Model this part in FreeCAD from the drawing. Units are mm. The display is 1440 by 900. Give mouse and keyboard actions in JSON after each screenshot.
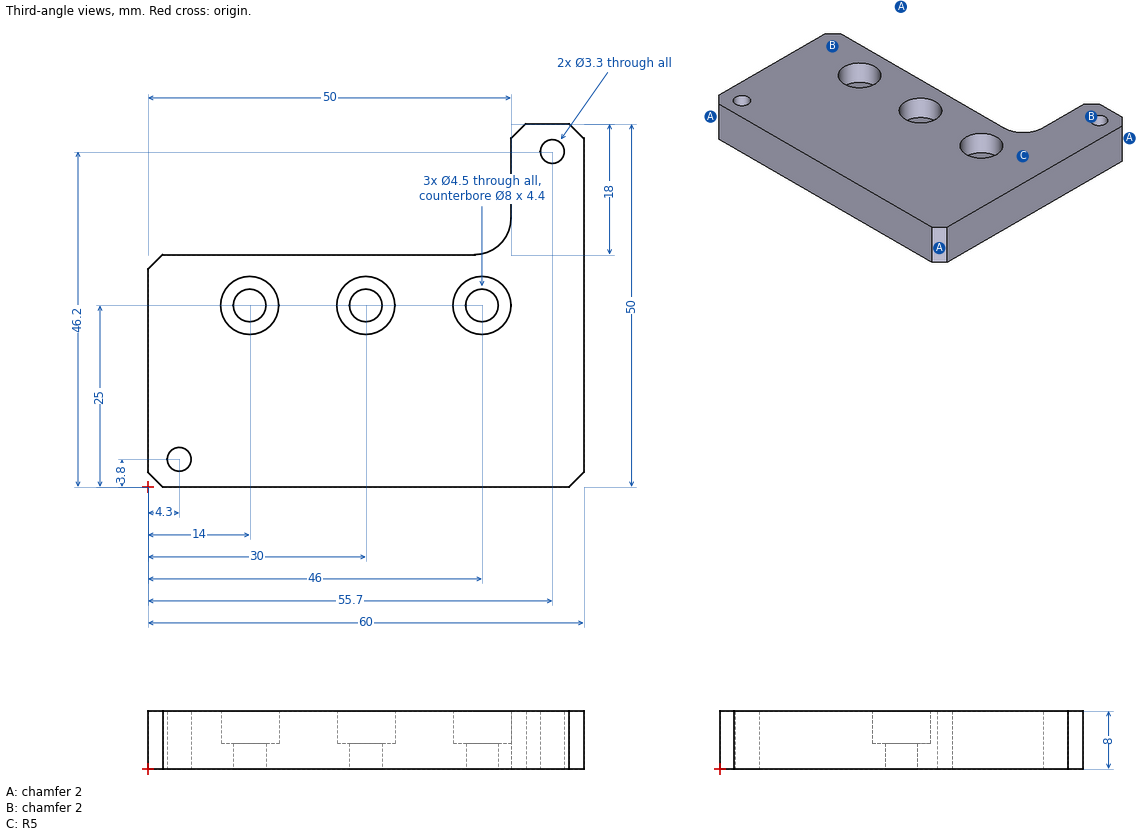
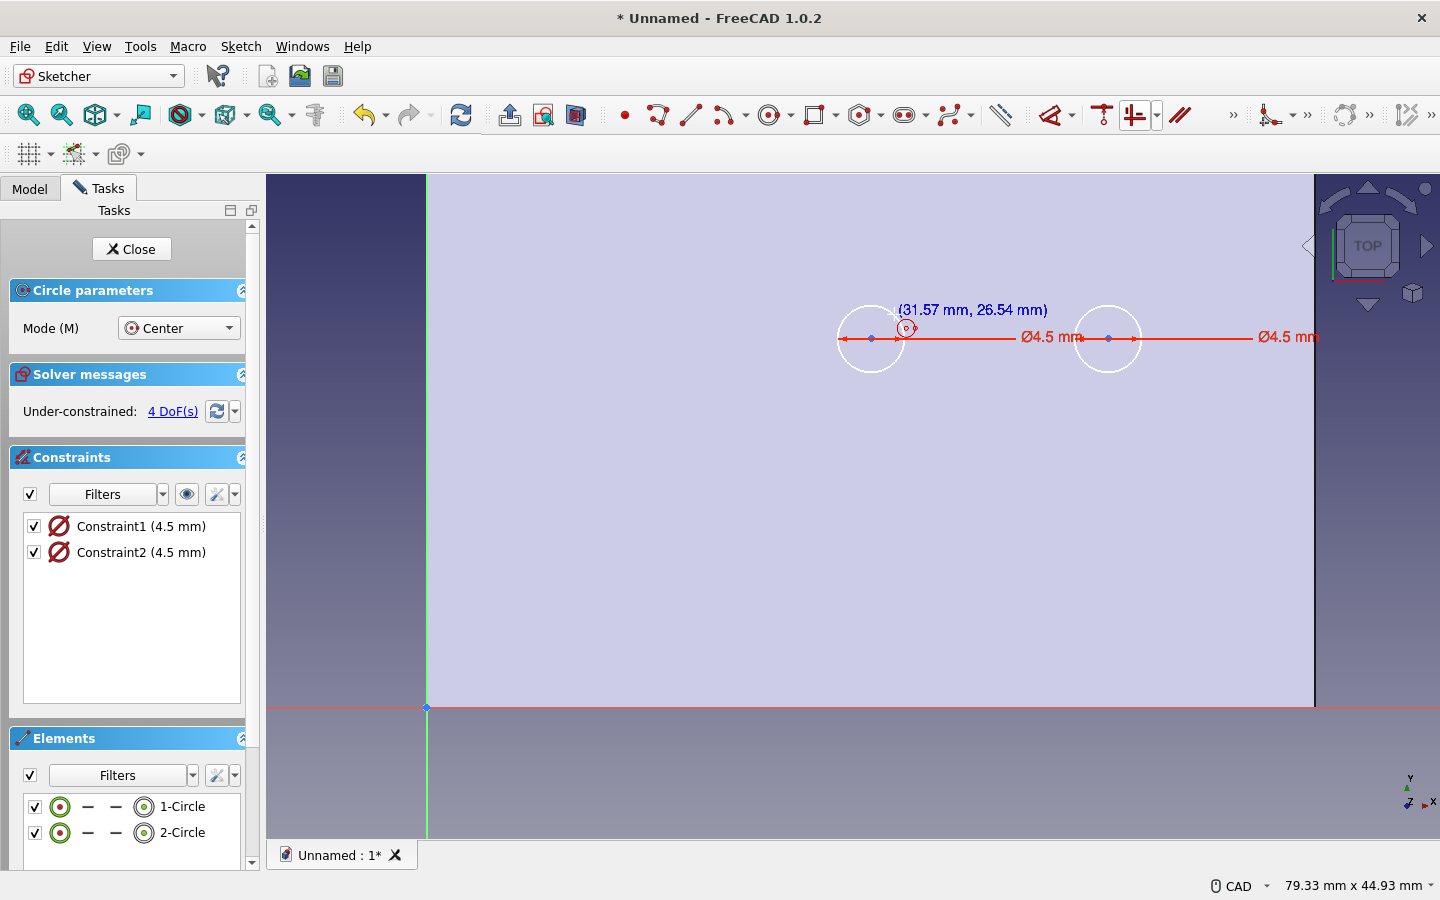
{"action": "left_click", "coordinate": [634, 338]}
{"action": "mouse_move", "coordinate": [658, 314]}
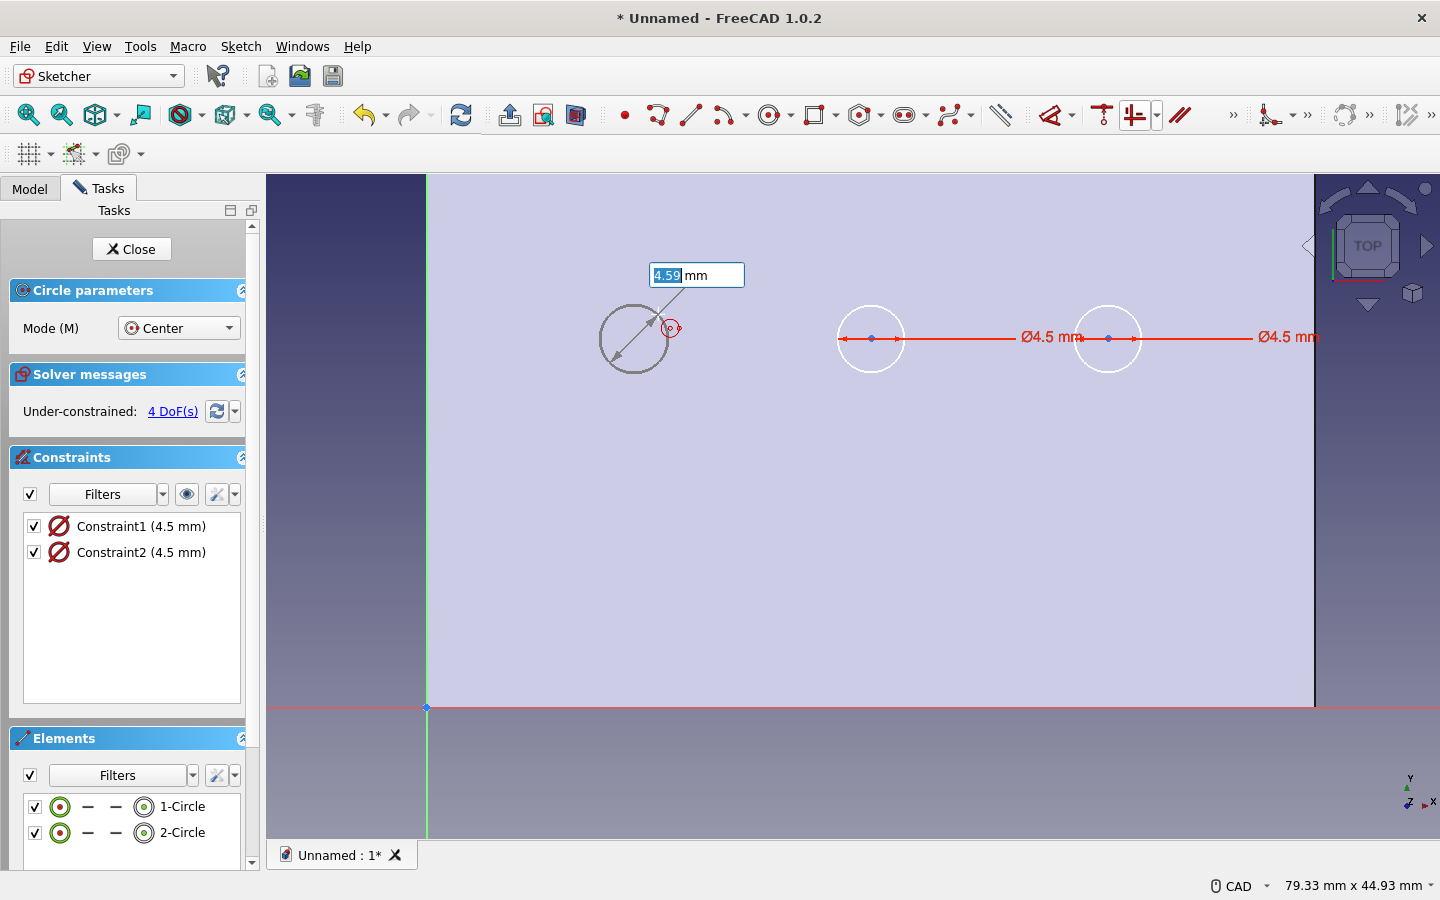
{"action": "type", "text": "4.5"}
{"action": "key", "text": "Return"}
{"action": "key", "text": "Escape"}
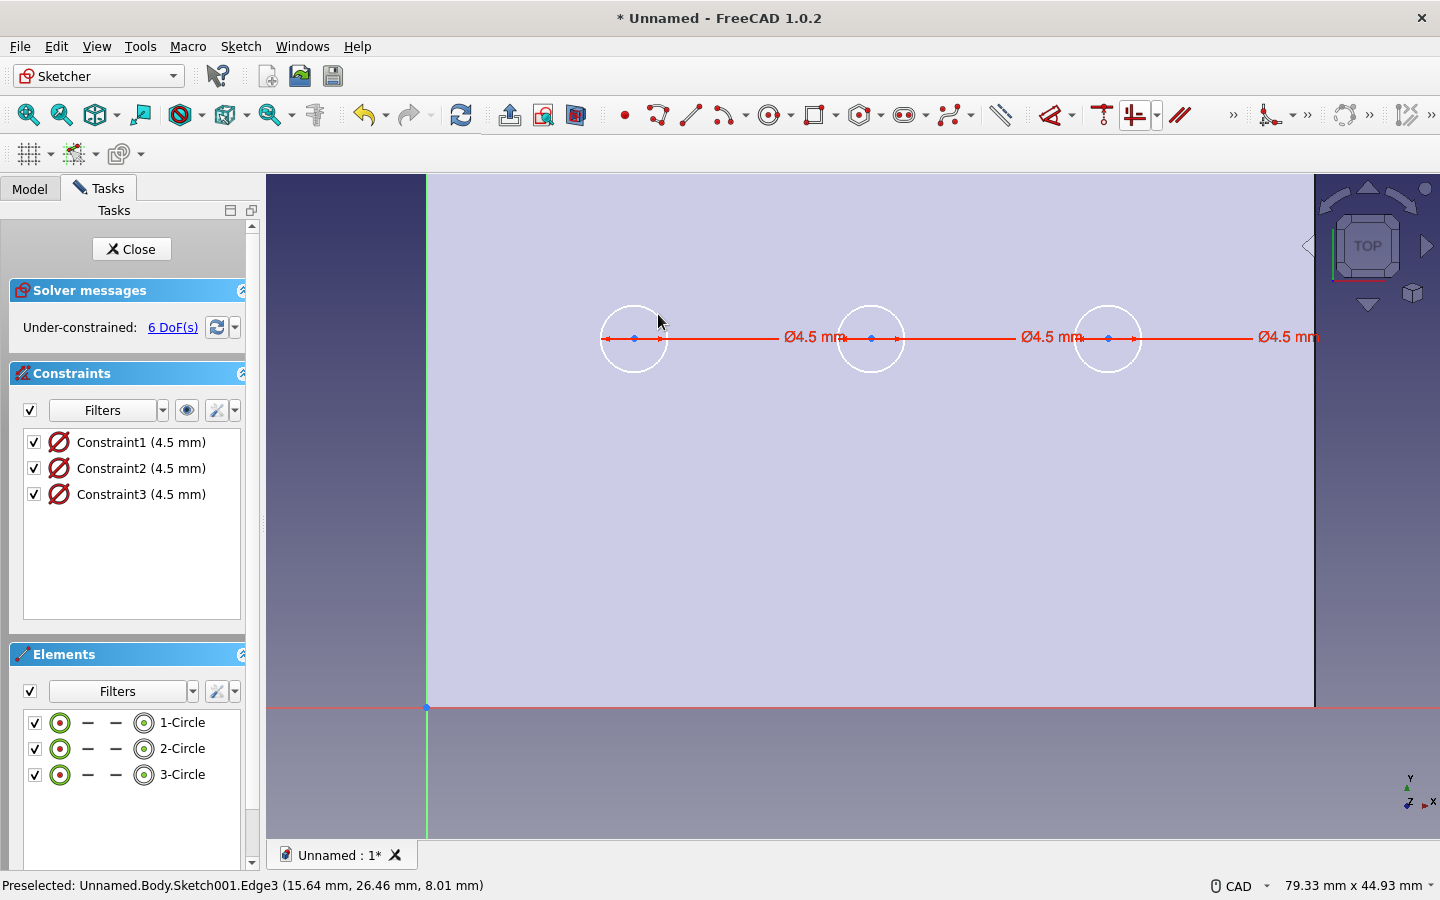
{"action": "left_click", "coordinate": [1108, 339]}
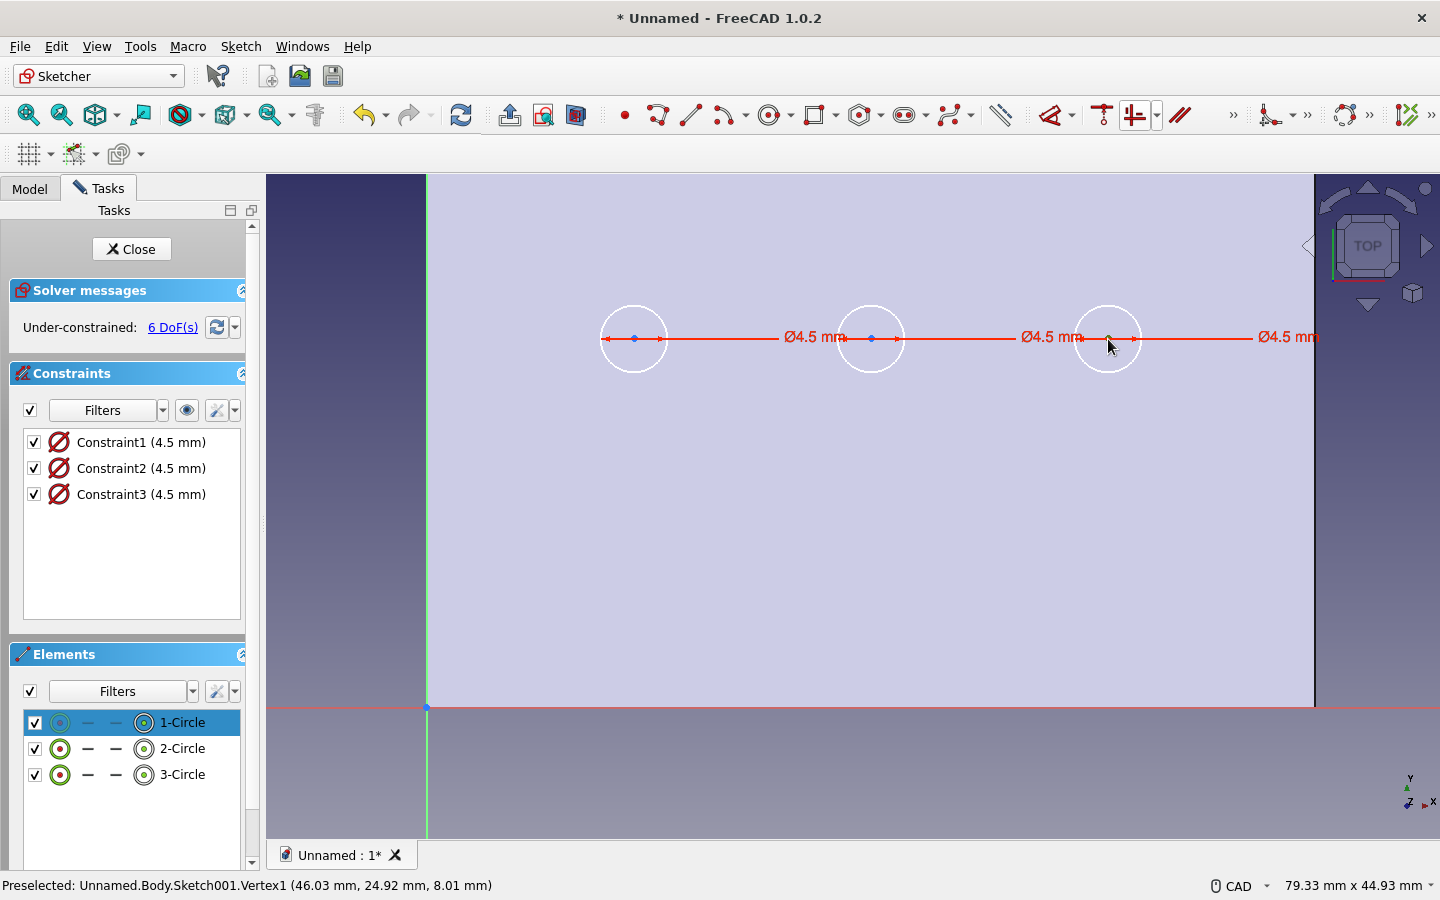
{"action": "left_click", "coordinate": [871, 339]}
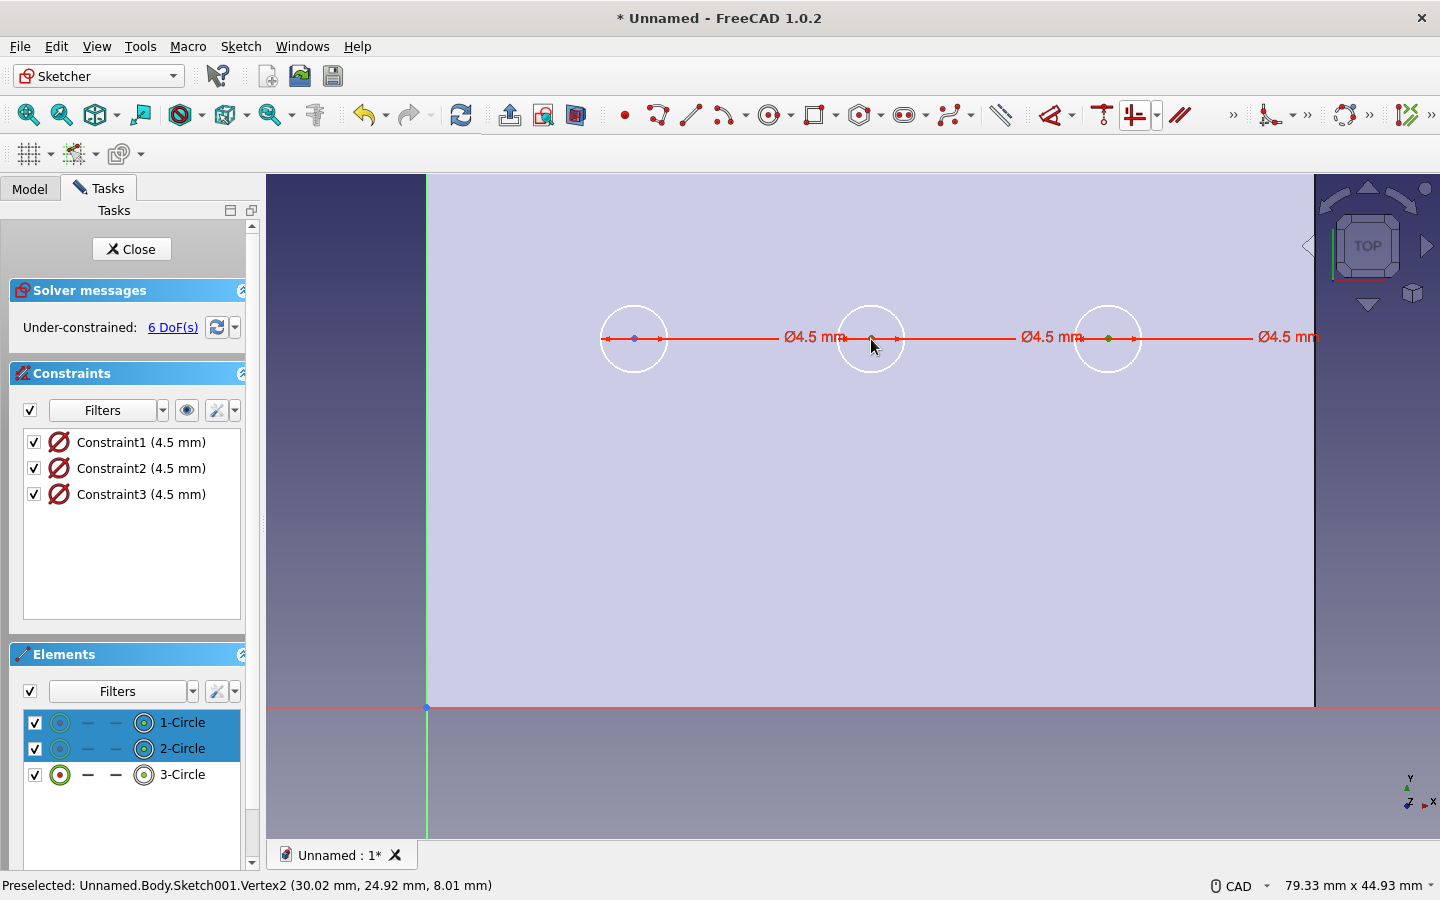
{"action": "left_click", "coordinate": [1156, 116]}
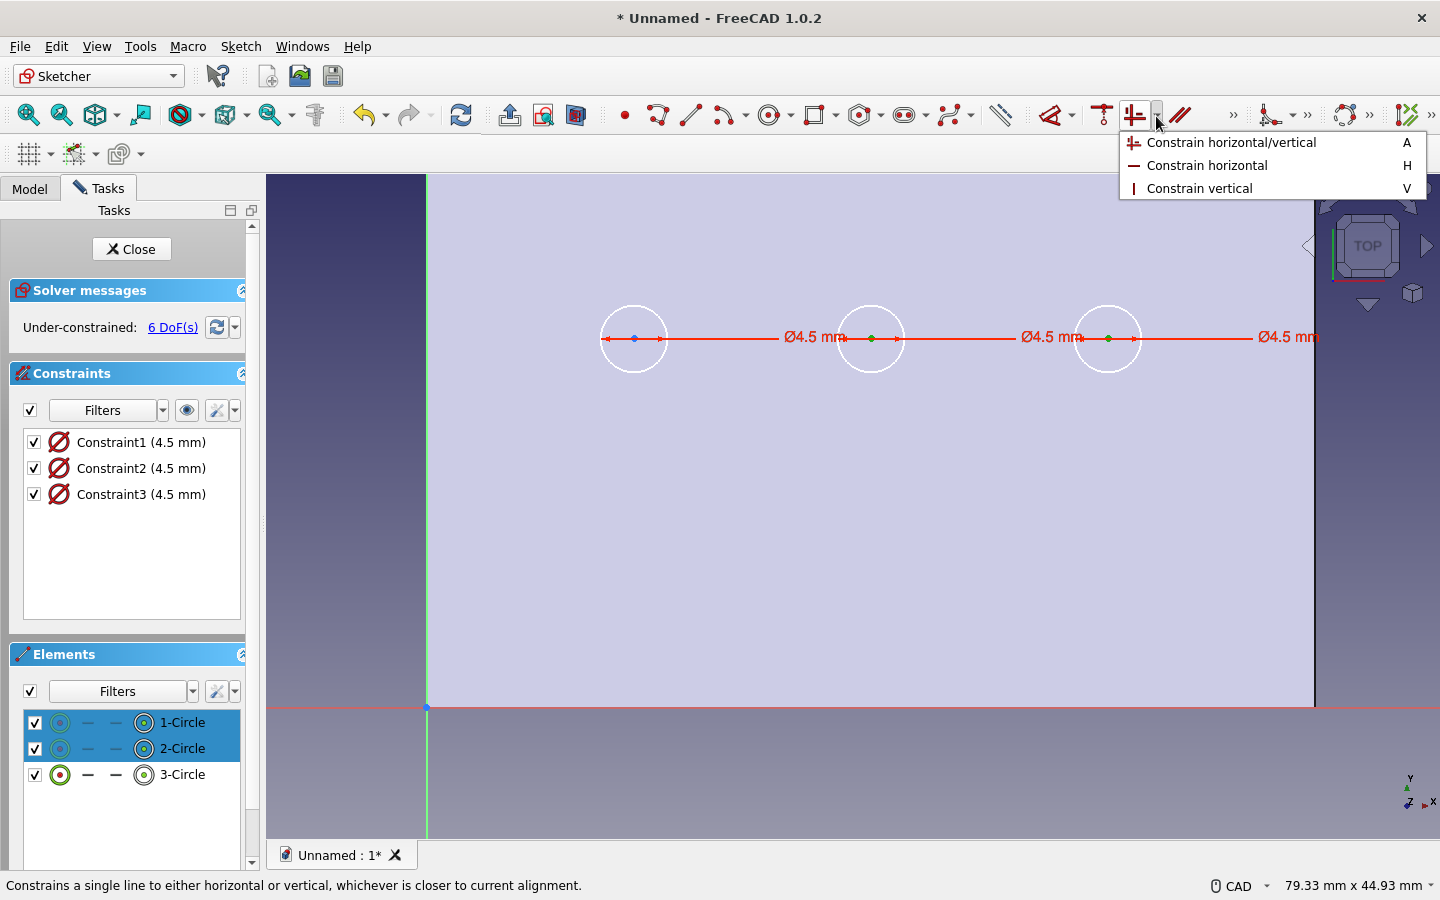
{"action": "left_click", "coordinate": [1273, 166]}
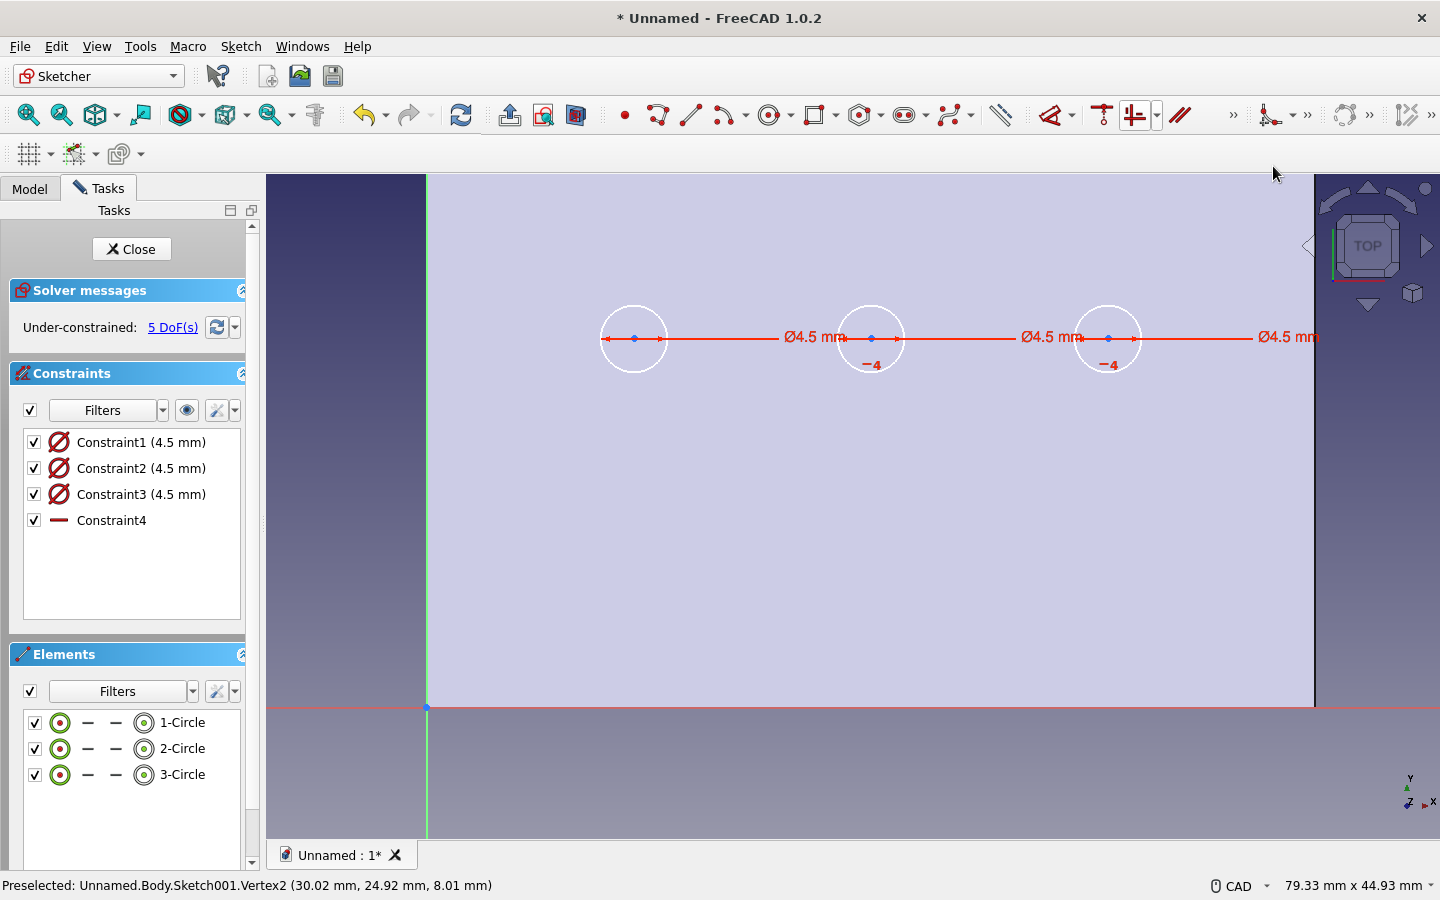
{"action": "left_click", "coordinate": [871, 339]}